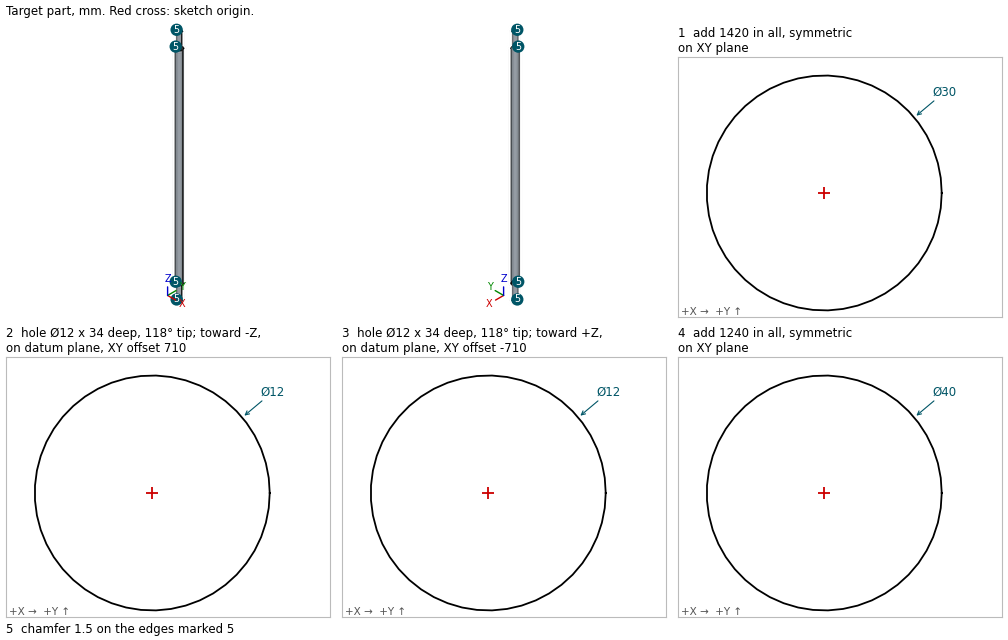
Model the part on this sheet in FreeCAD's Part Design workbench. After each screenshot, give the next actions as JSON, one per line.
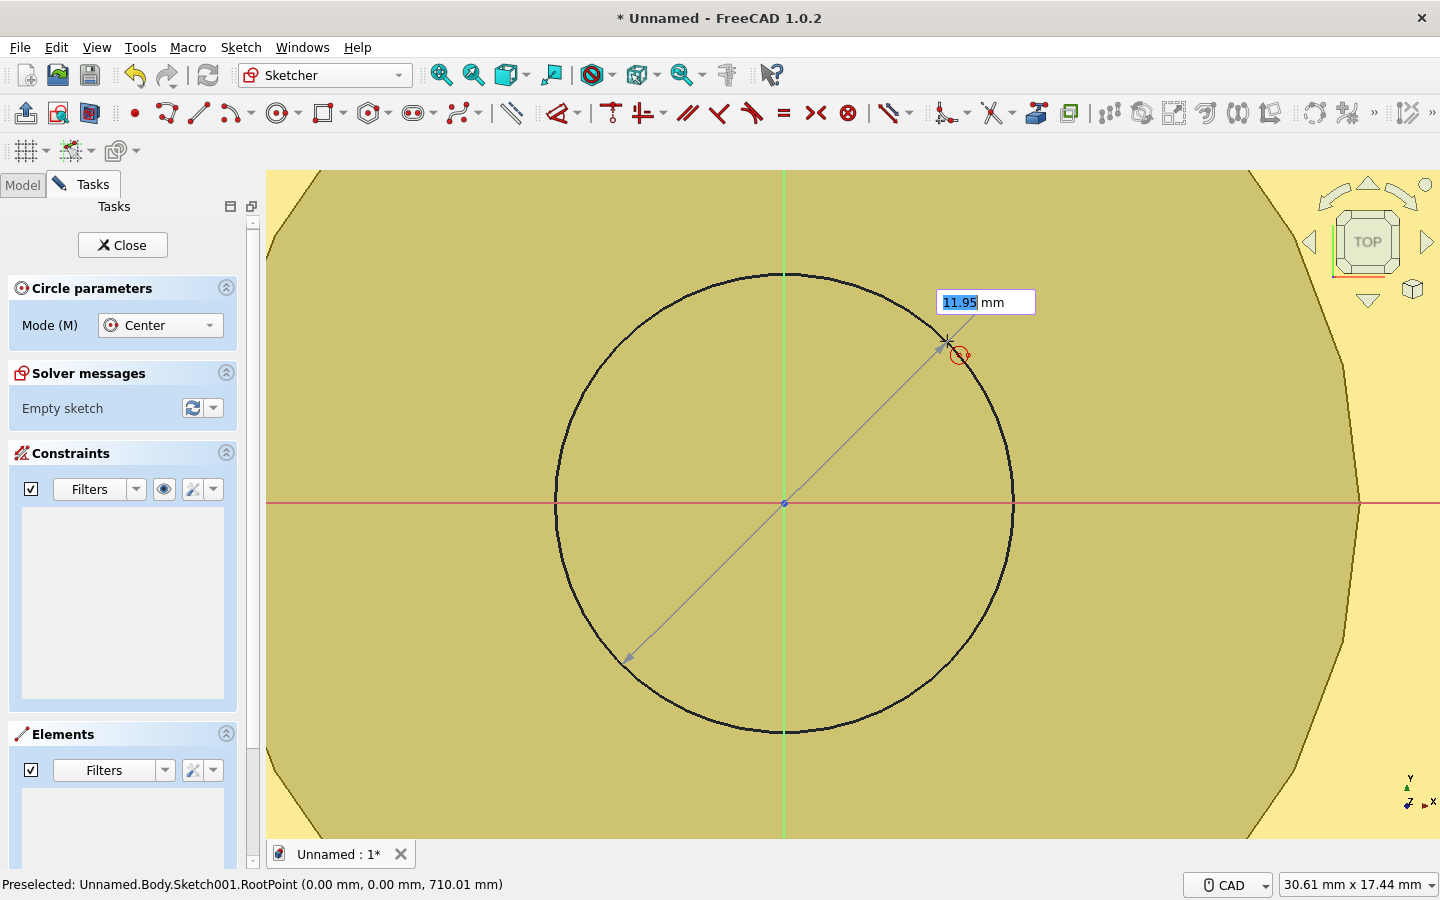
{"action": "type", "text": "12"}
{"action": "key", "text": "Return"}
{"action": "key", "text": "Escape"}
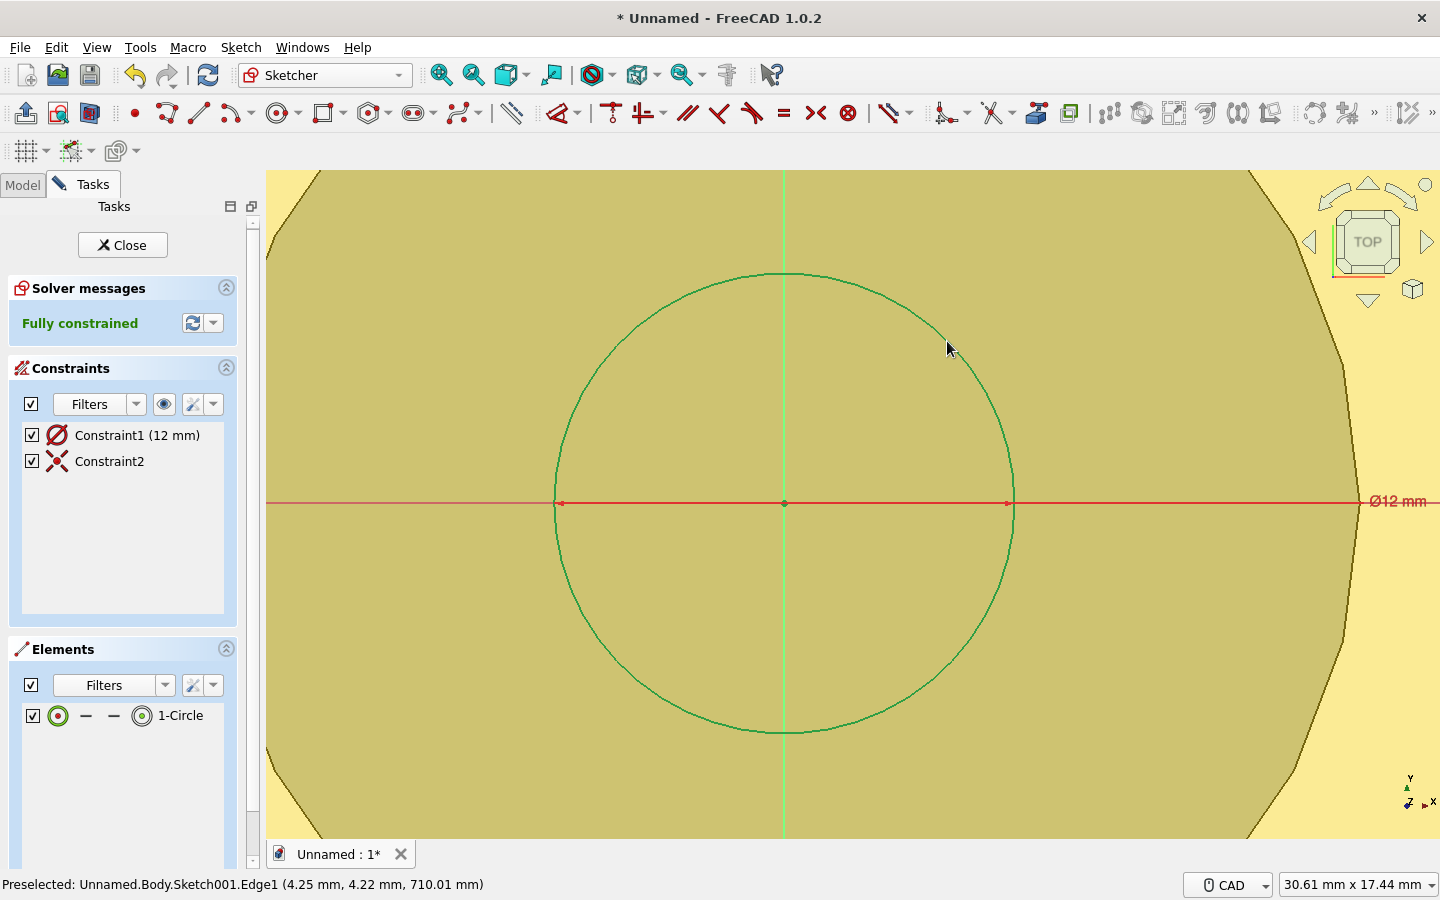
{"action": "left_click", "coordinate": [123, 245]}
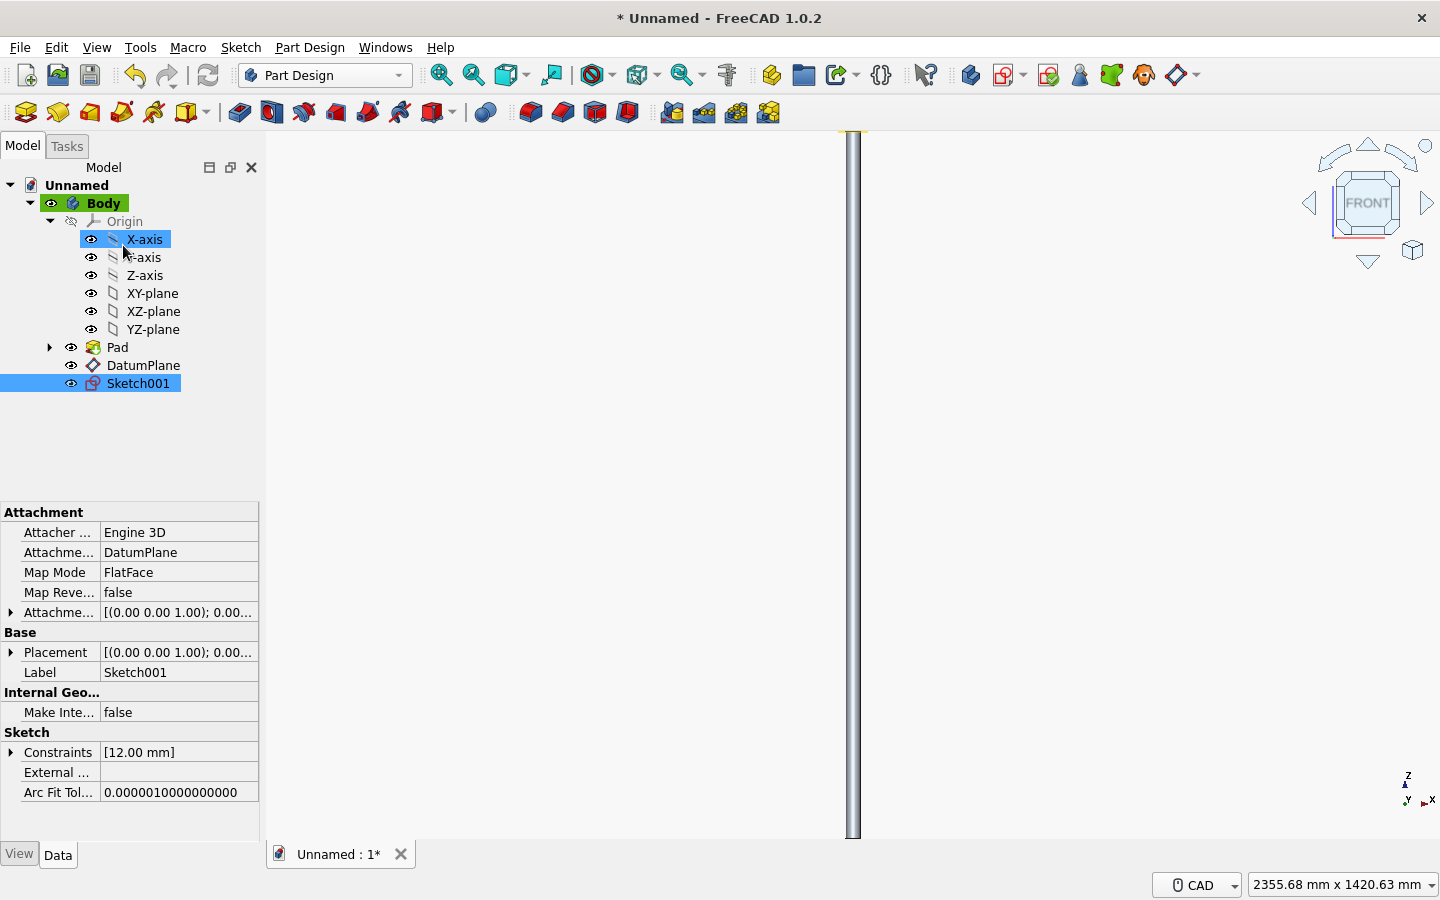
{"action": "left_click", "coordinate": [272, 112]}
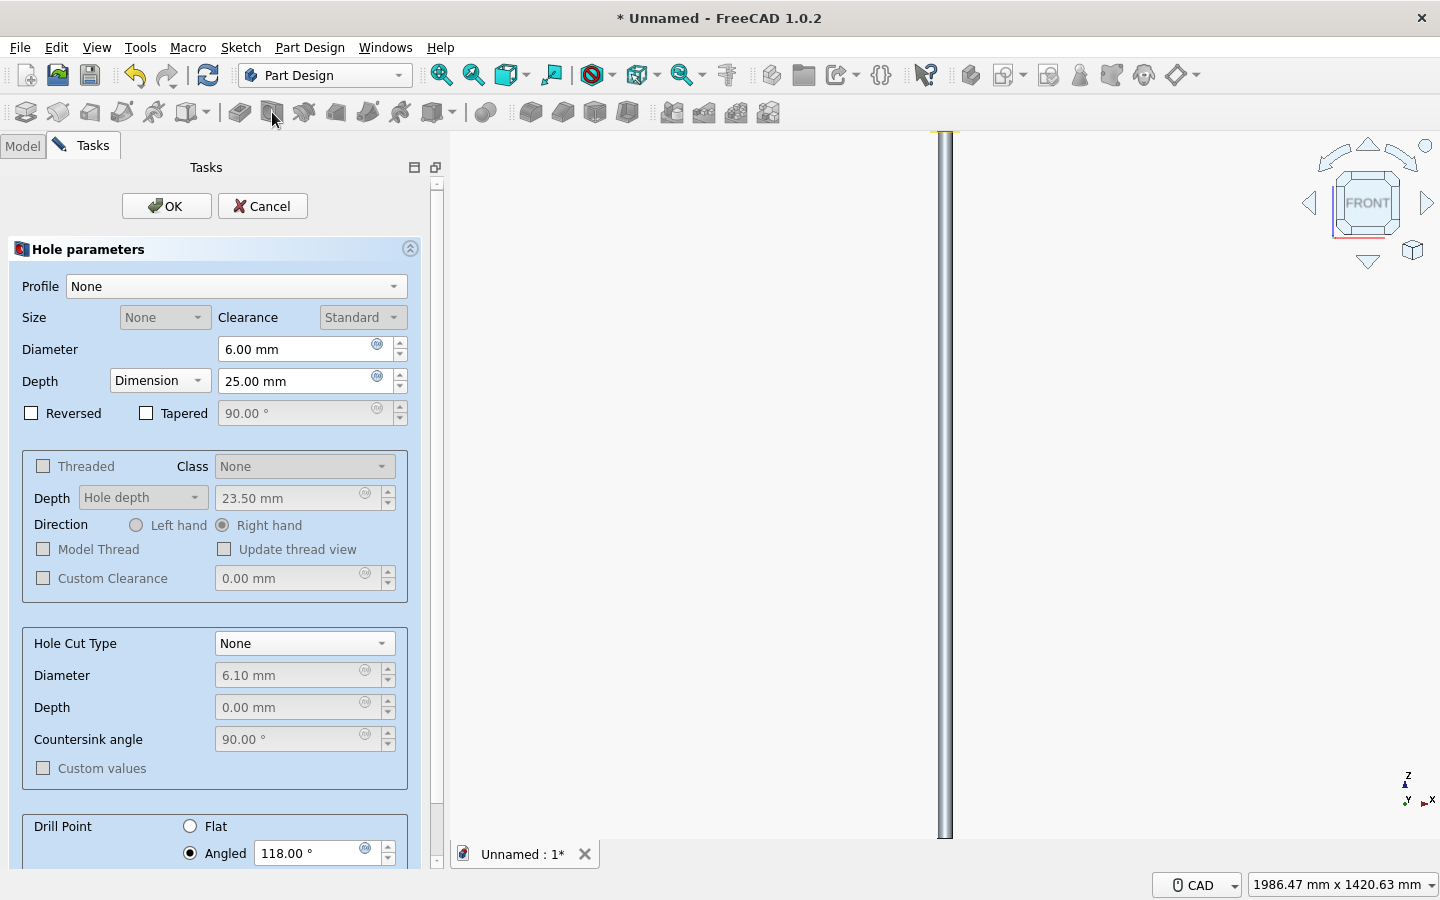
{"action": "triple_click", "coordinate": [305, 349]}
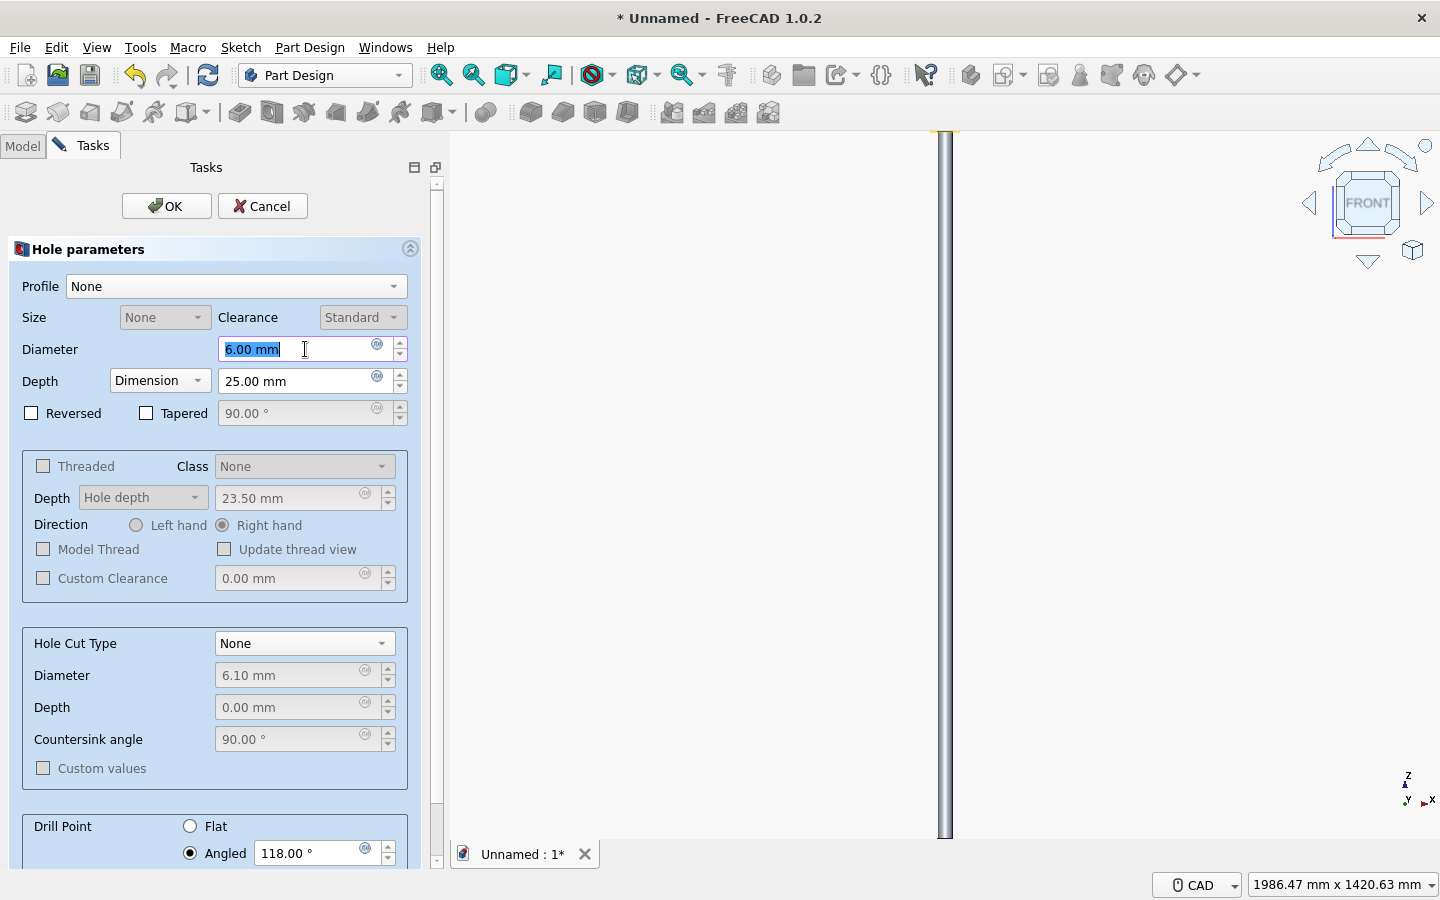
{"action": "type", "text": "12"}
{"action": "key", "text": "Tab"}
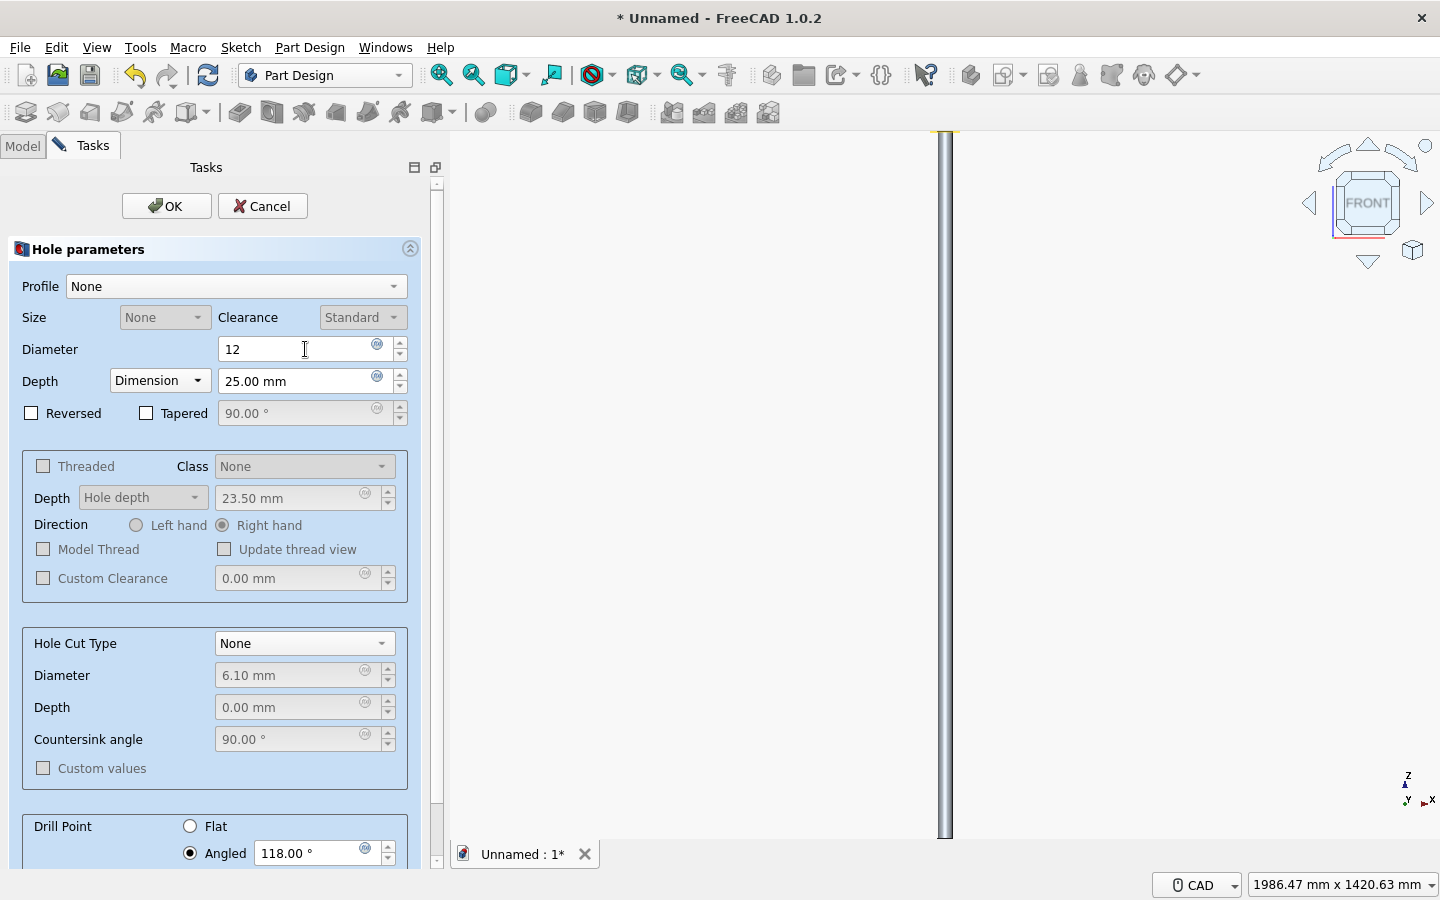
{"action": "triple_click", "coordinate": [305, 381]}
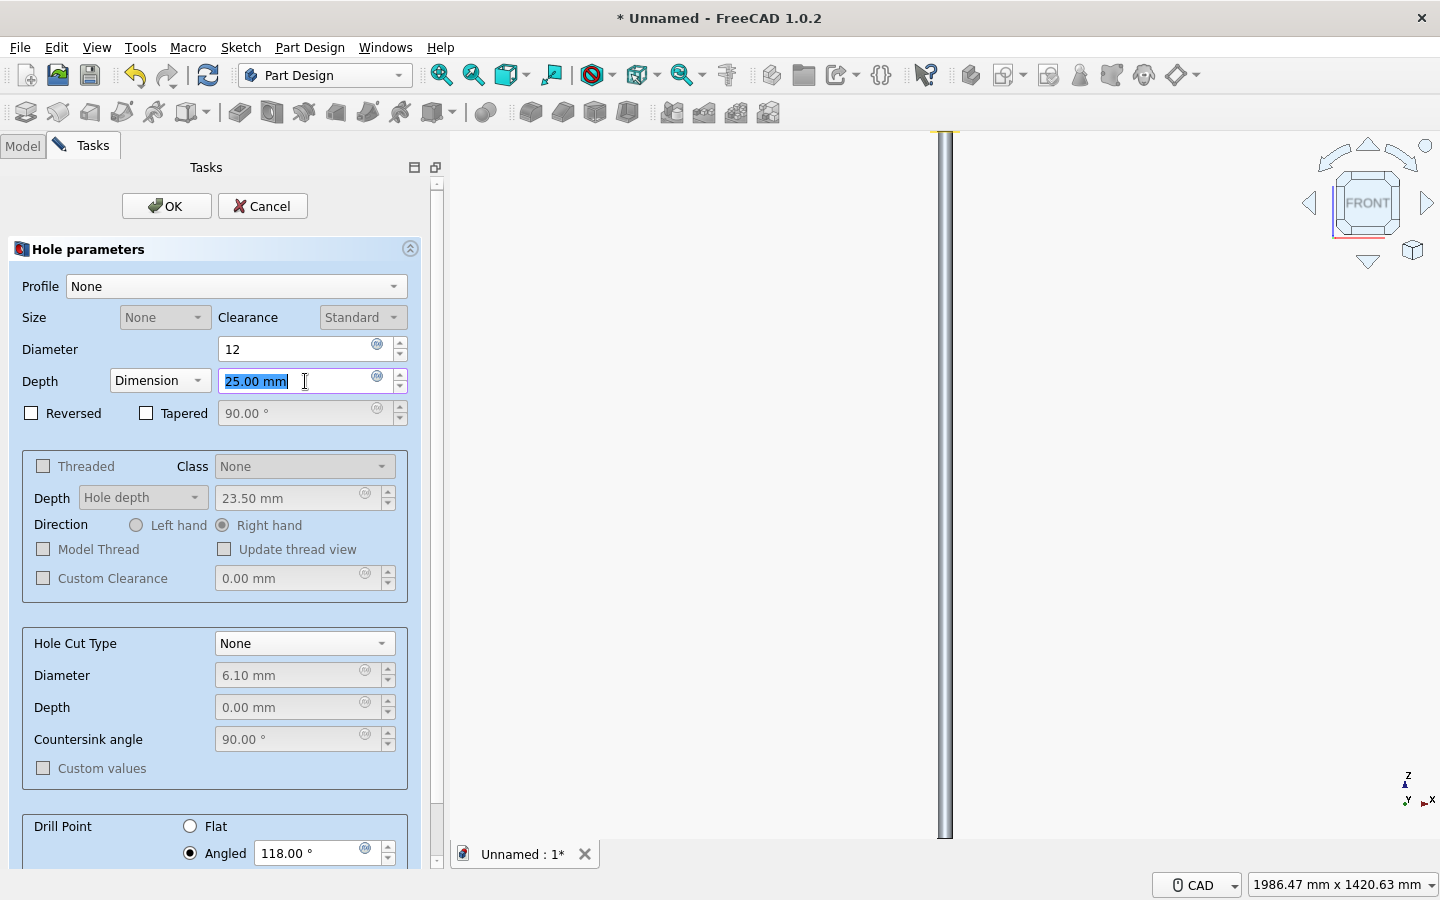
{"action": "type", "text": "34"}
{"action": "key", "text": "Tab"}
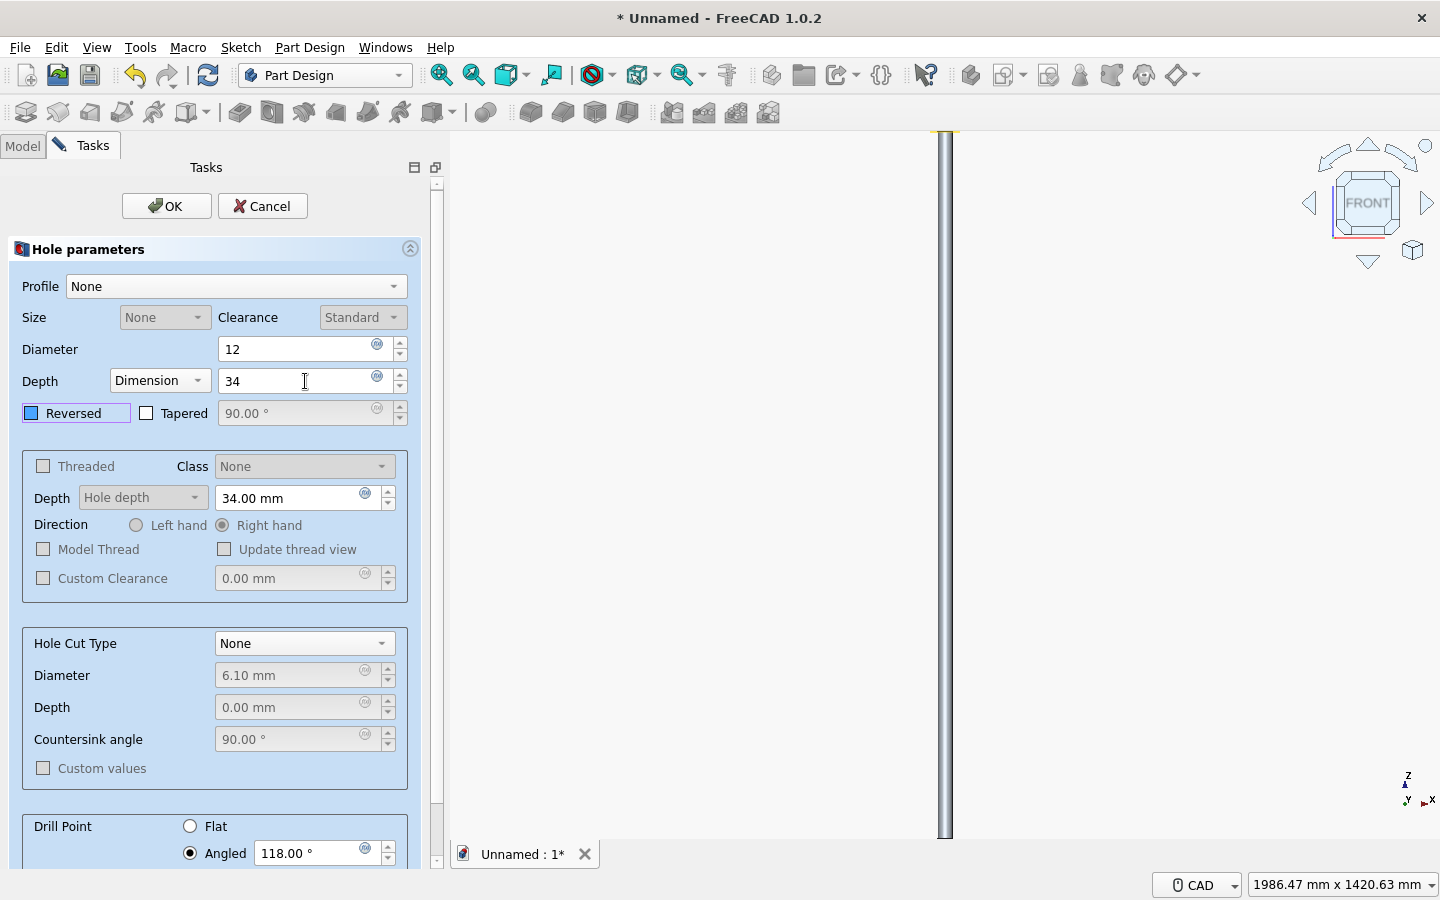
{"action": "left_click", "coordinate": [167, 206]}